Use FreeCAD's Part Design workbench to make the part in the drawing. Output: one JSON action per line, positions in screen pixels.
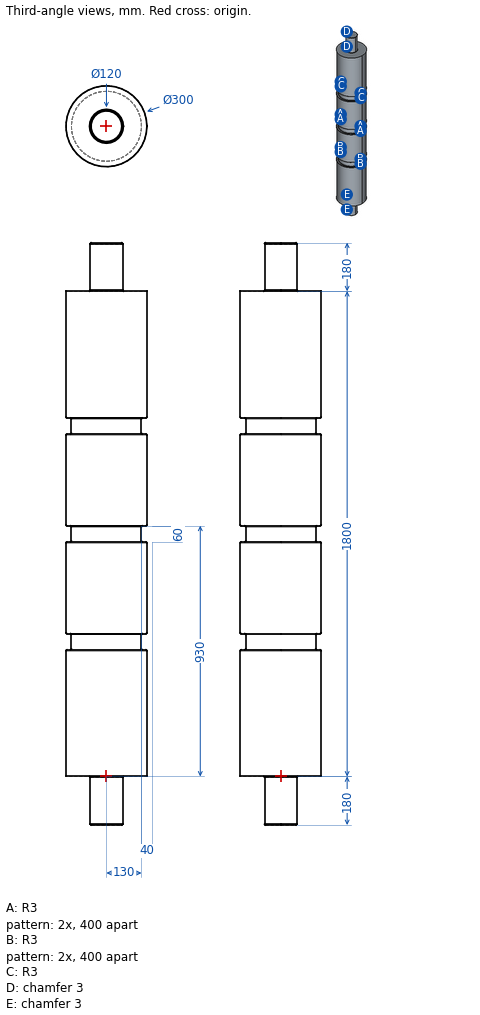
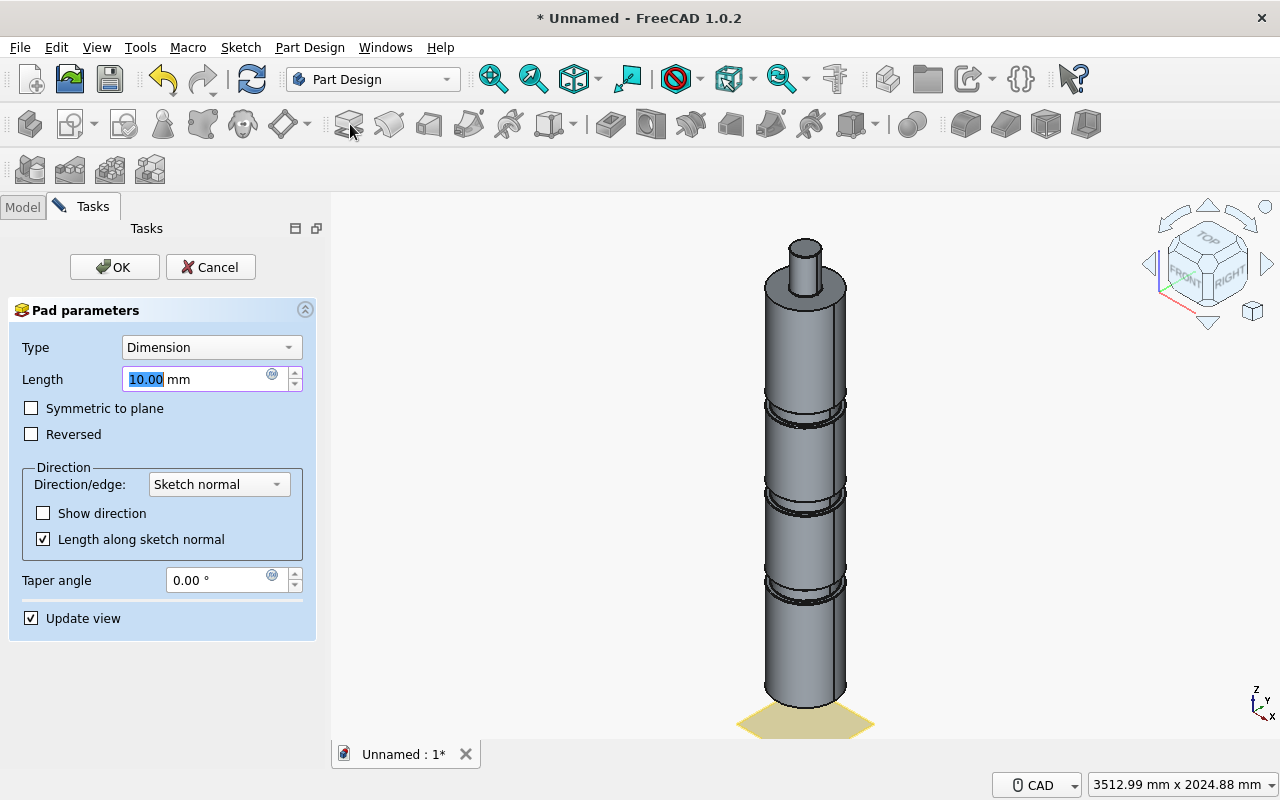
{"action": "type", "text": "180"}
{"action": "key", "text": "Tab"}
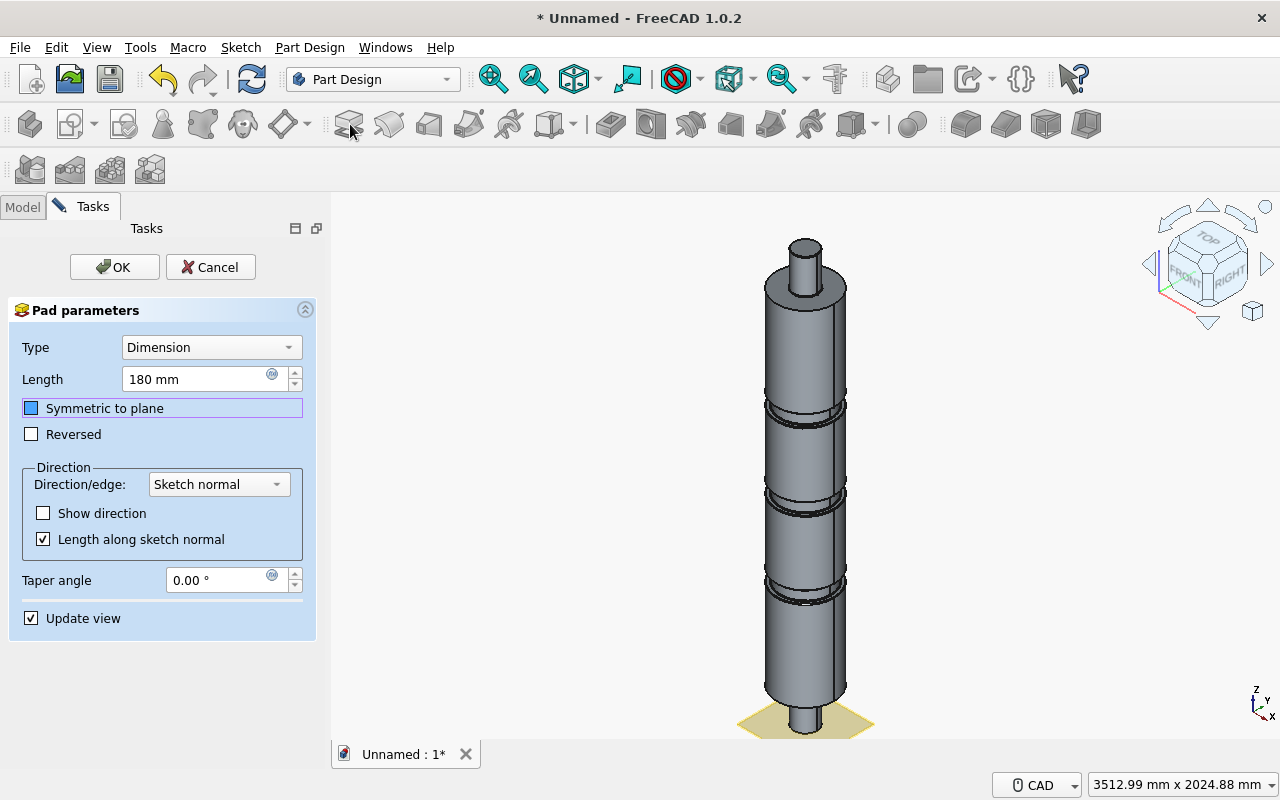
{"action": "left_click", "coordinate": [115, 267]}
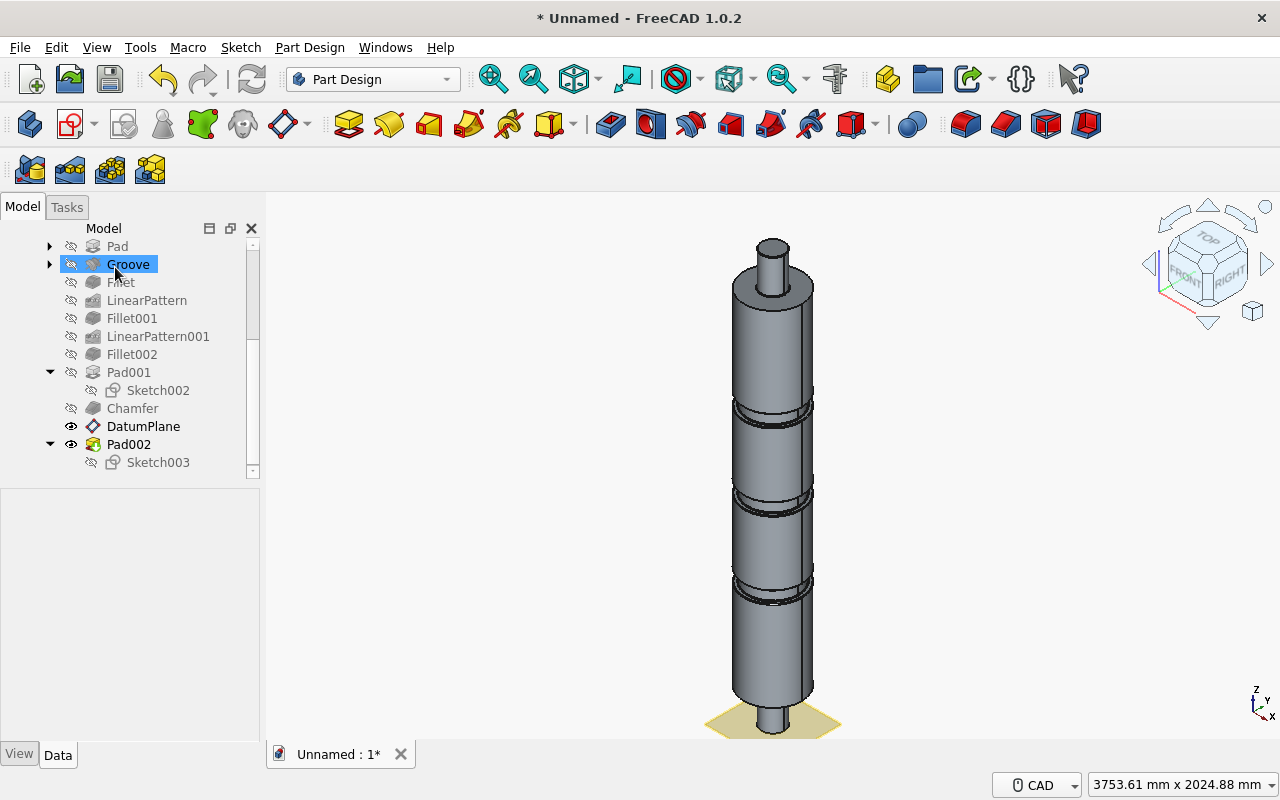
{"action": "left_click", "coordinate": [116, 426]}
{"action": "key", "text": "space"}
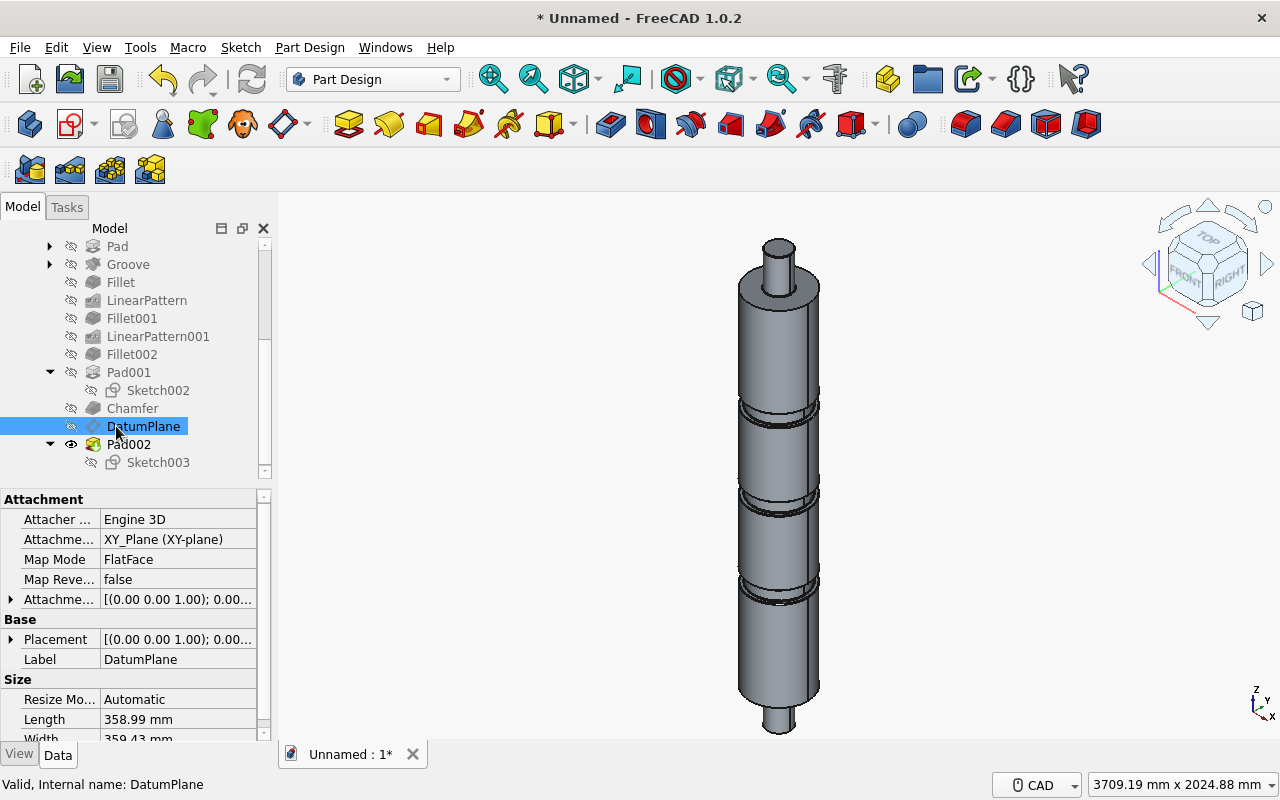
{"action": "left_click", "coordinate": [494, 80]}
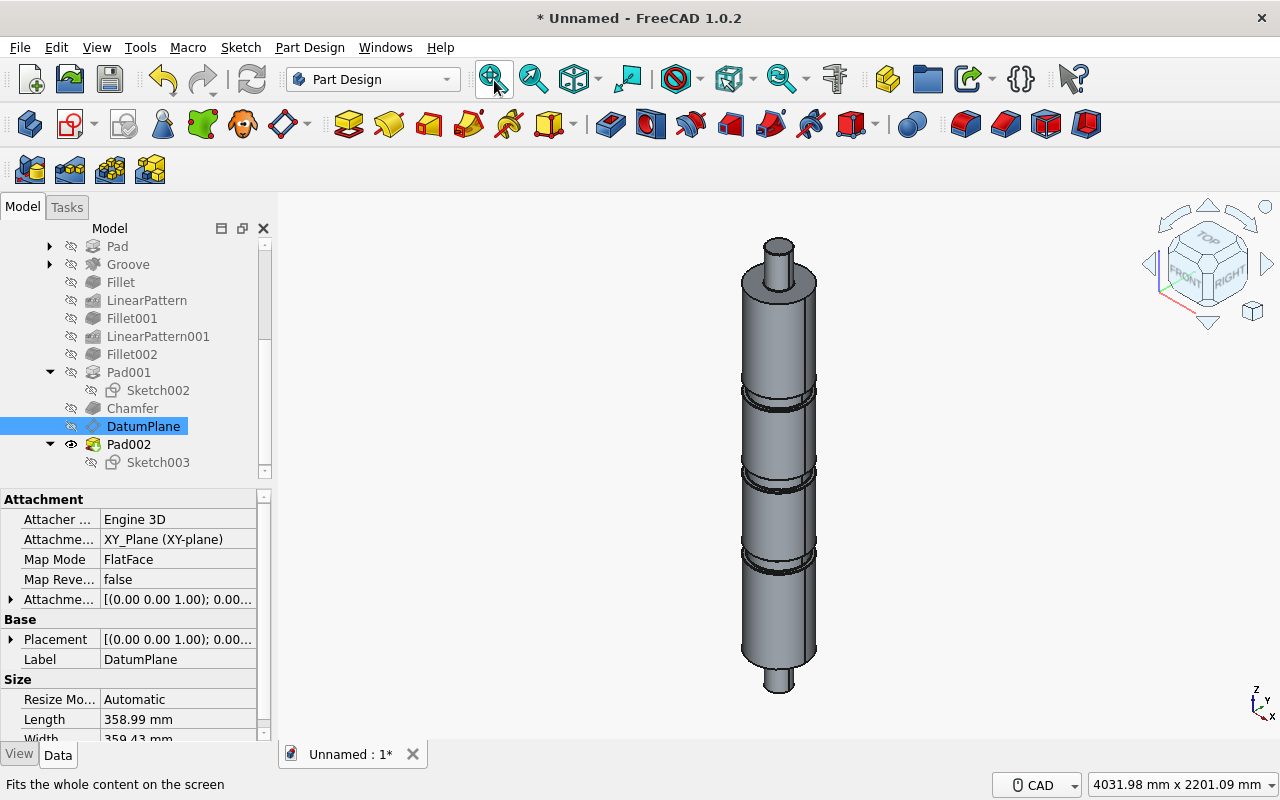
{"action": "left_click", "coordinate": [766, 688]}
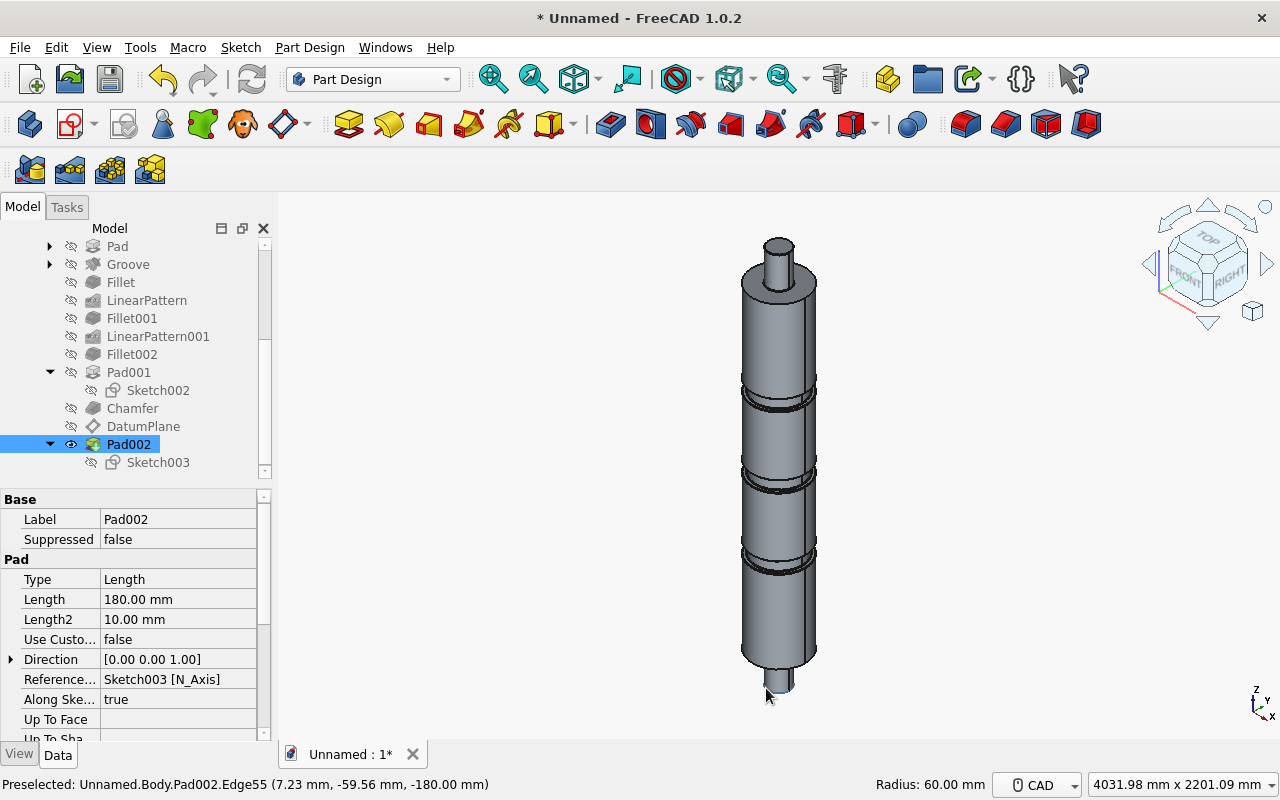
{"action": "key", "text": "2"}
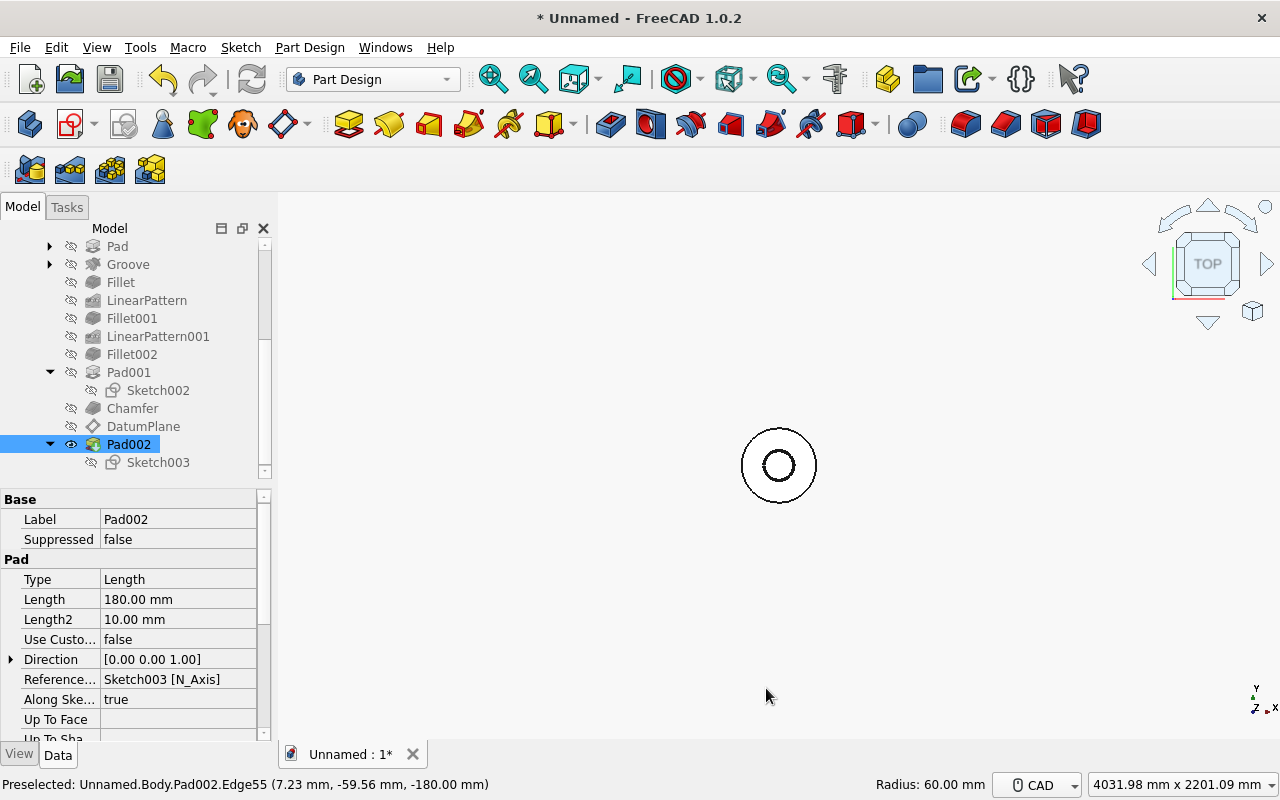
{"action": "left_click", "coordinate": [494, 80]}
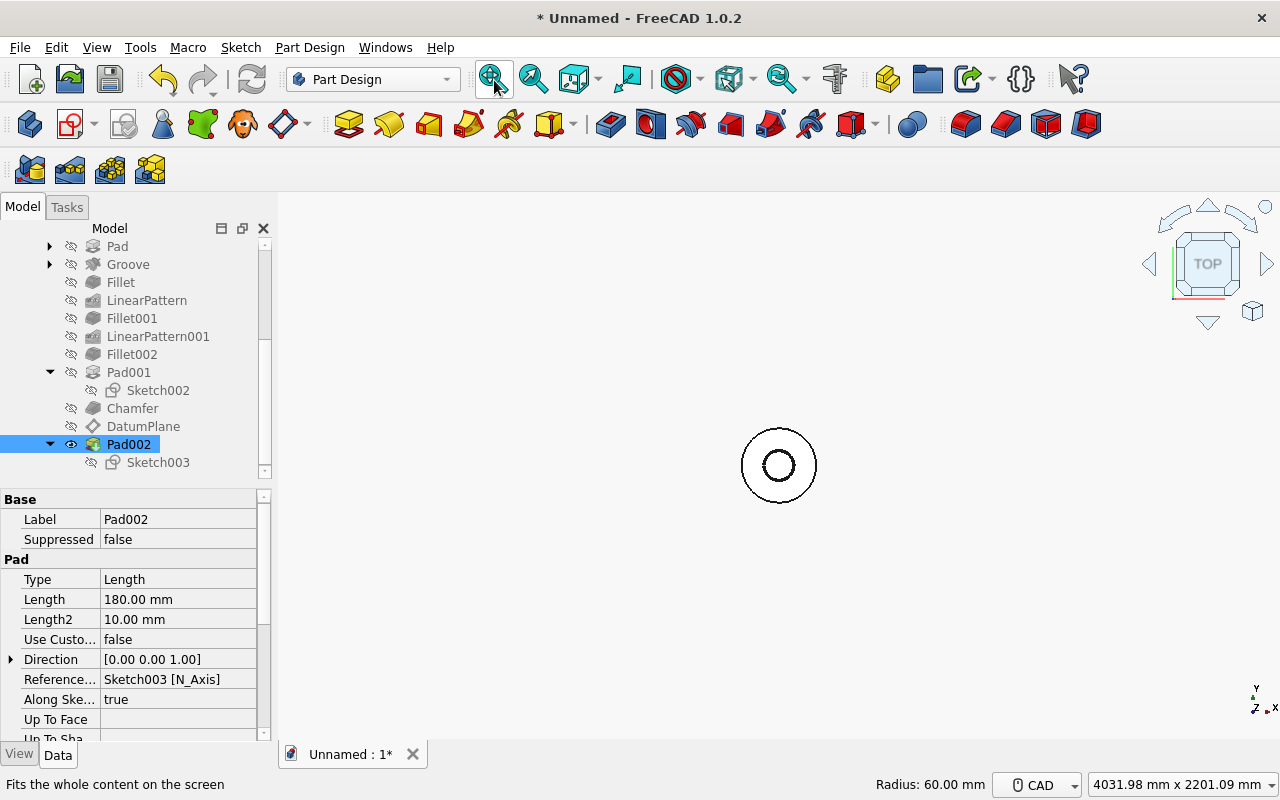
{"action": "key", "text": "0"}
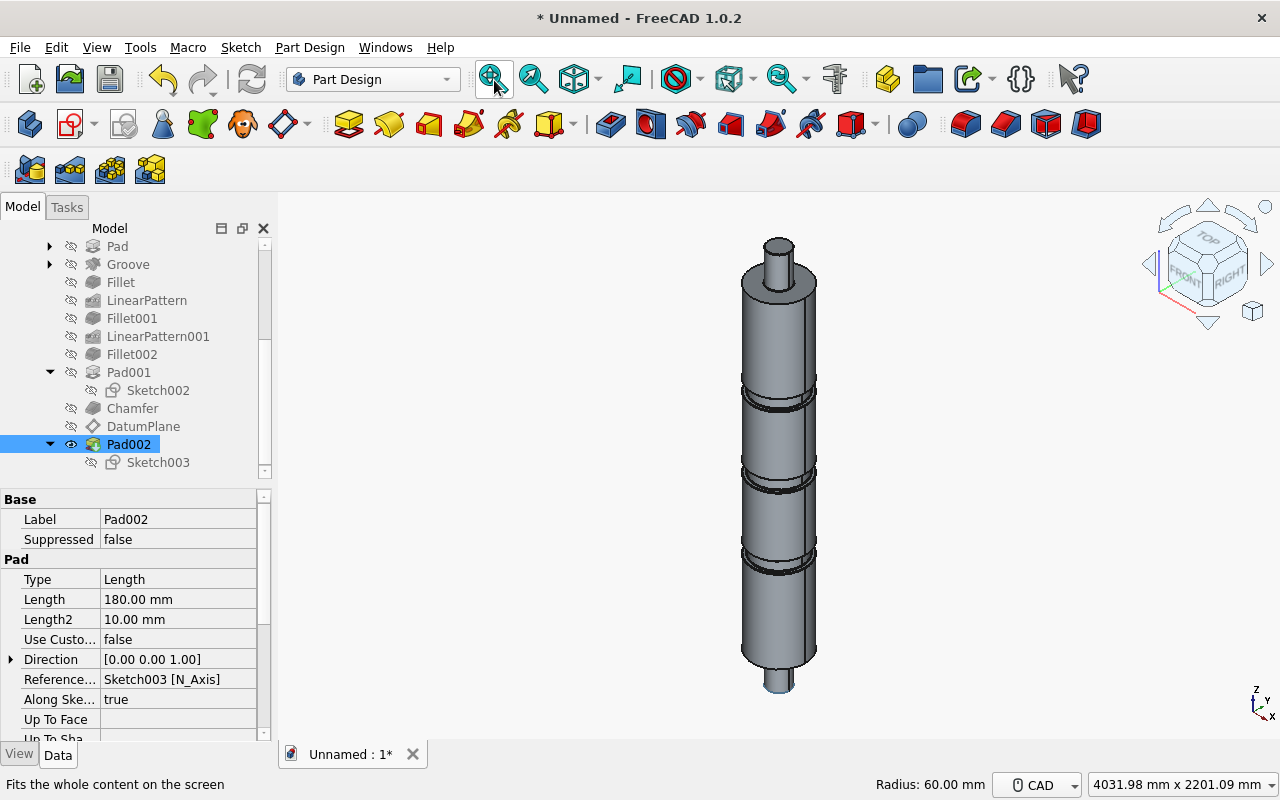
{"action": "key", "text": "1"}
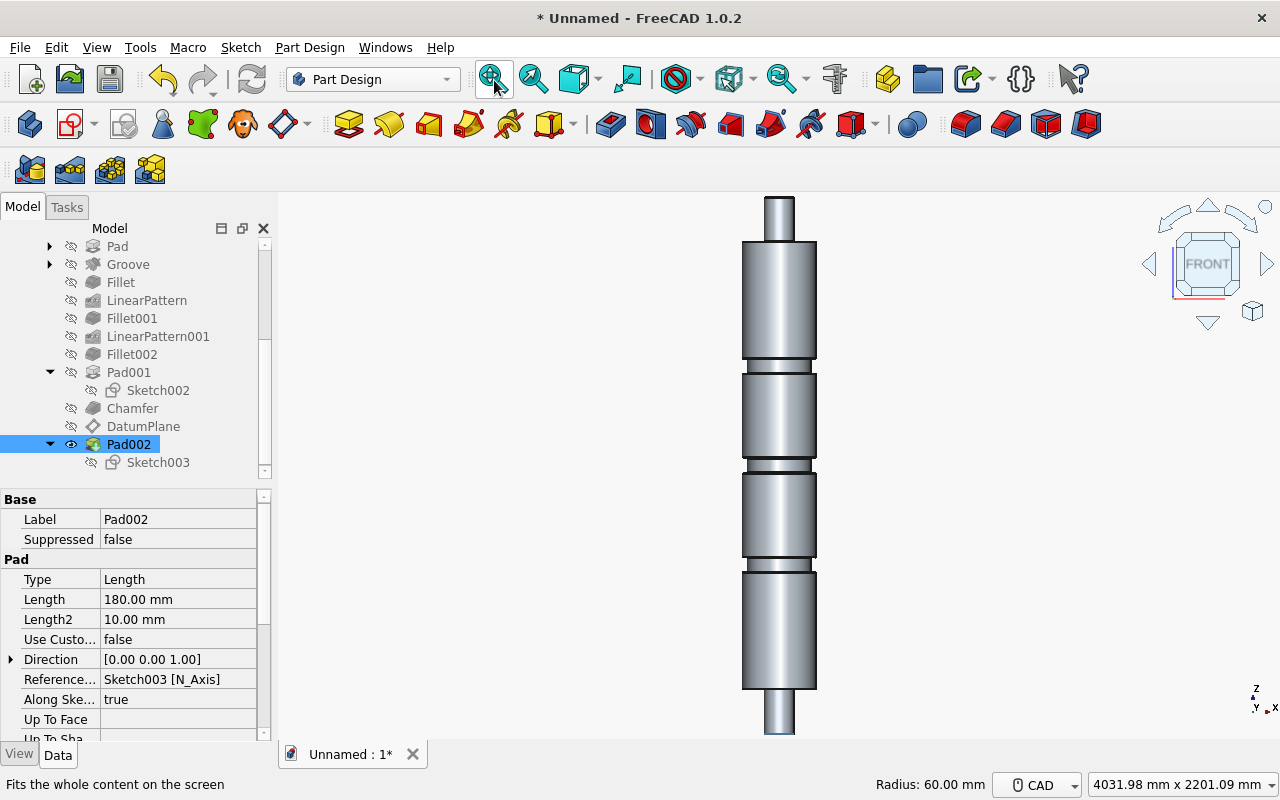
{"action": "key", "text": "3"}